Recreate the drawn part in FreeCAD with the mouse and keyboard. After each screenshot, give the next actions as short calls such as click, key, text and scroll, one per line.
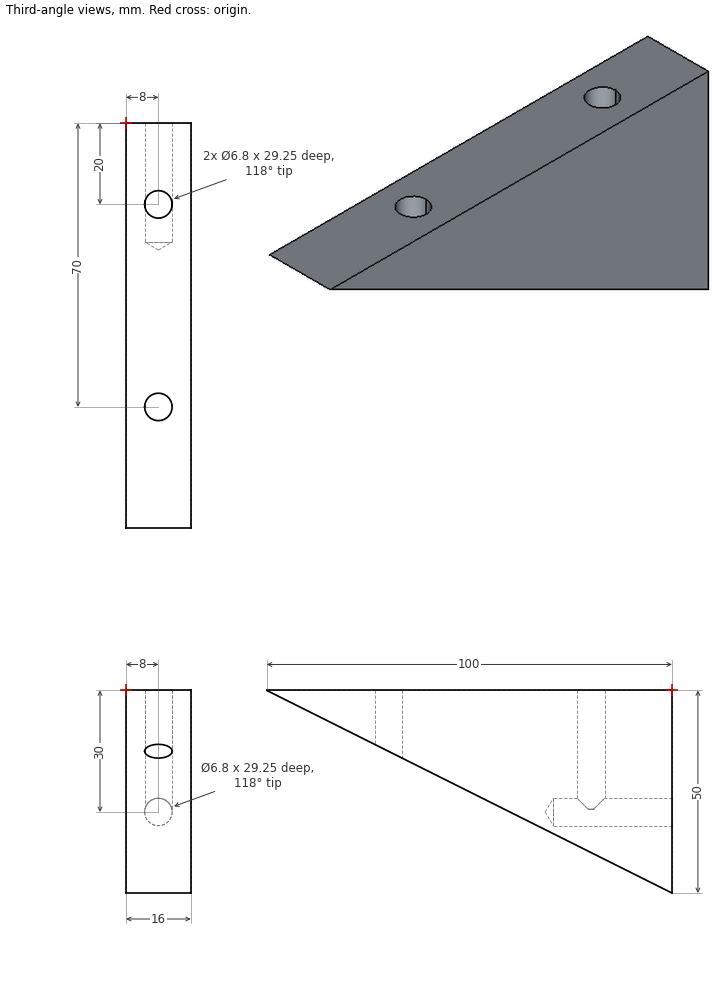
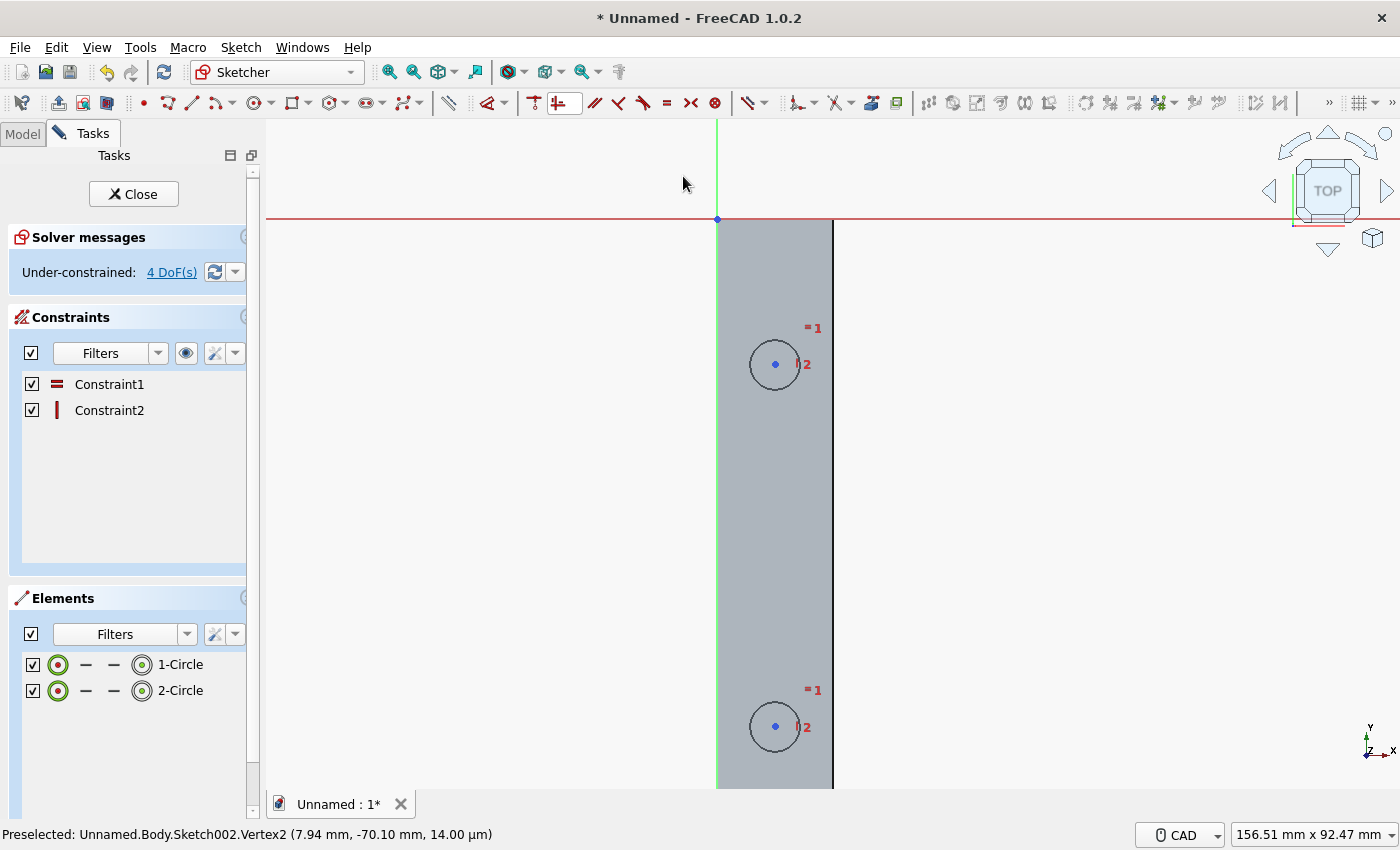
click(488, 104)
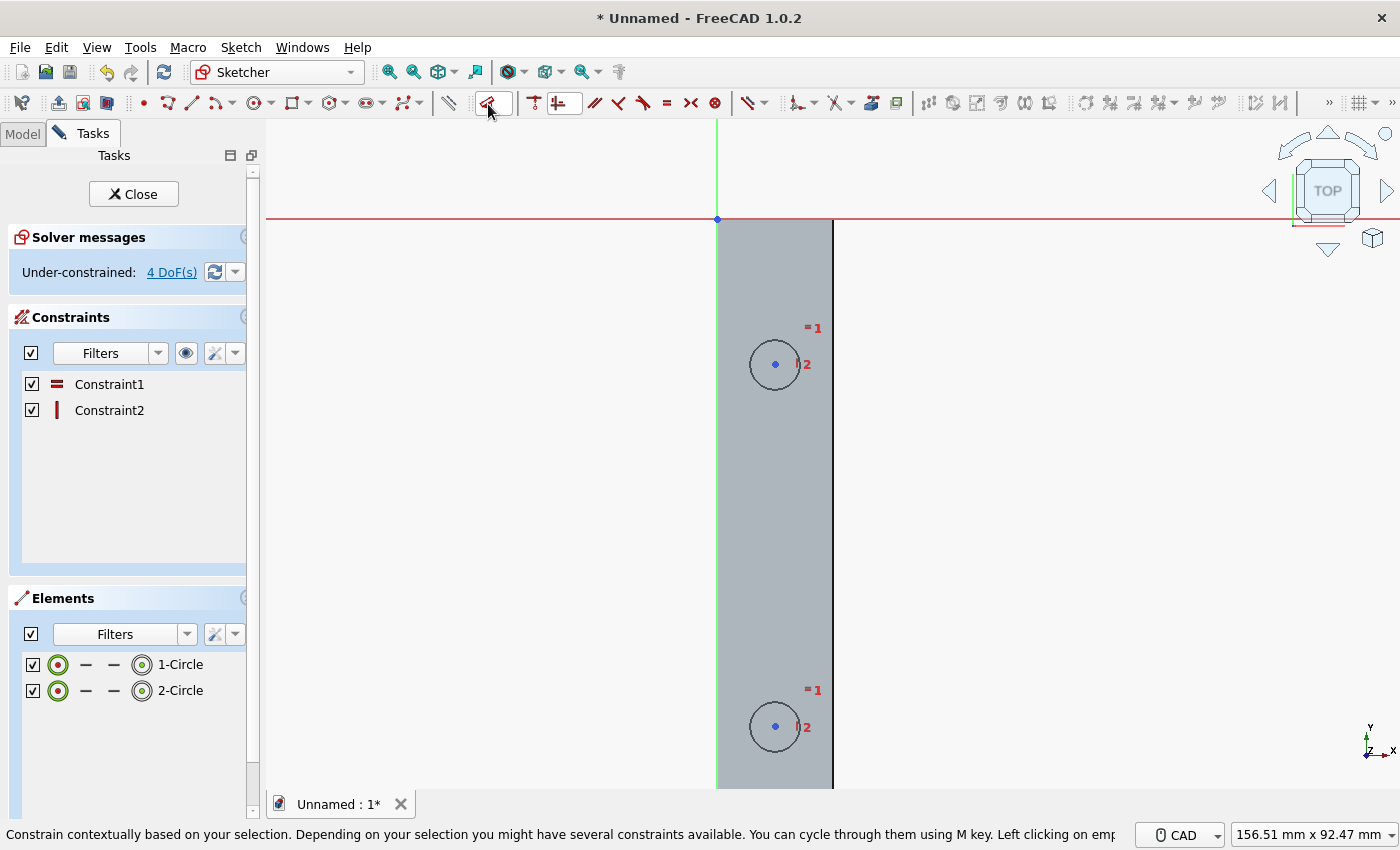
click(792, 347)
click(814, 324)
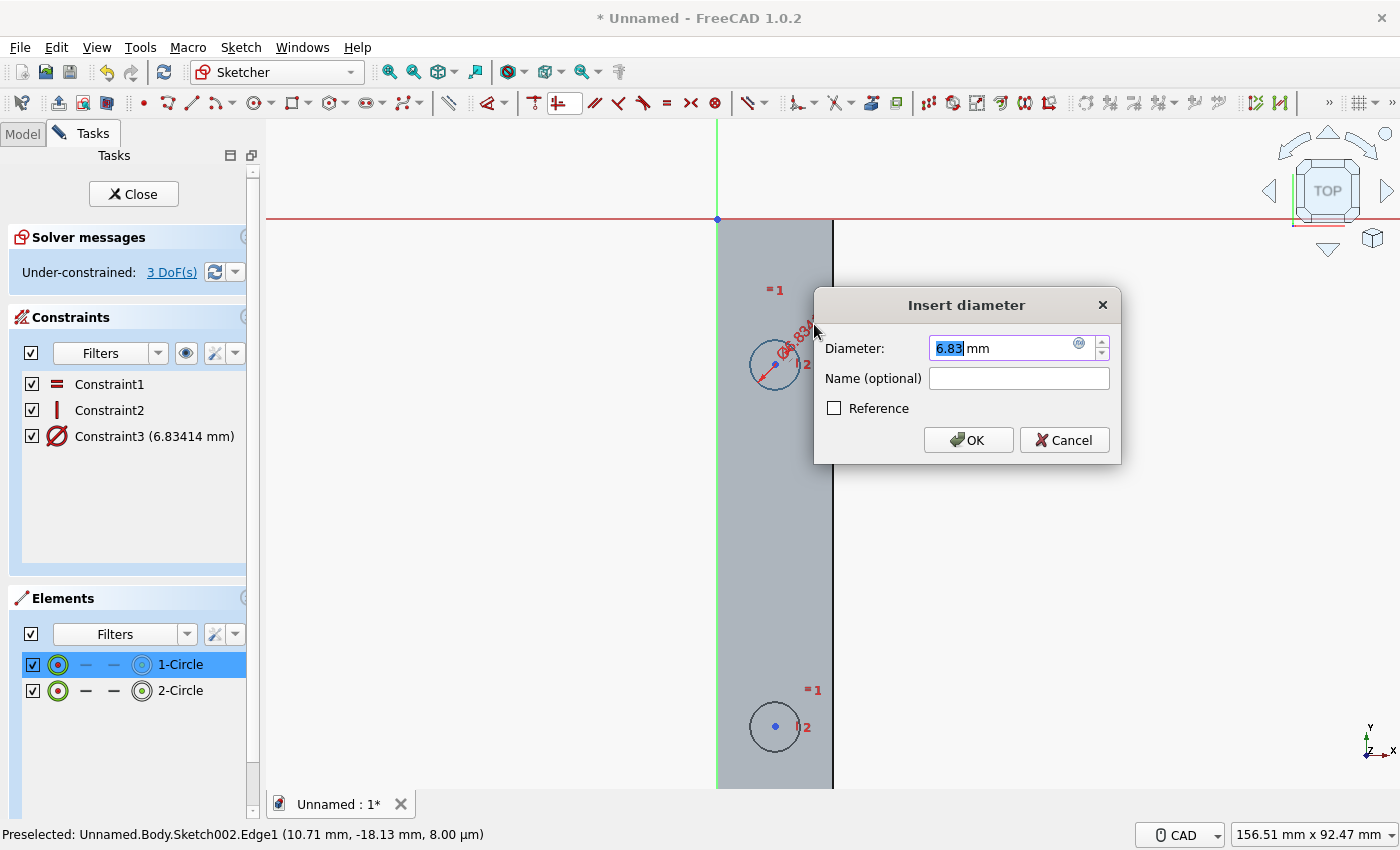
text(6.8)
key(Return)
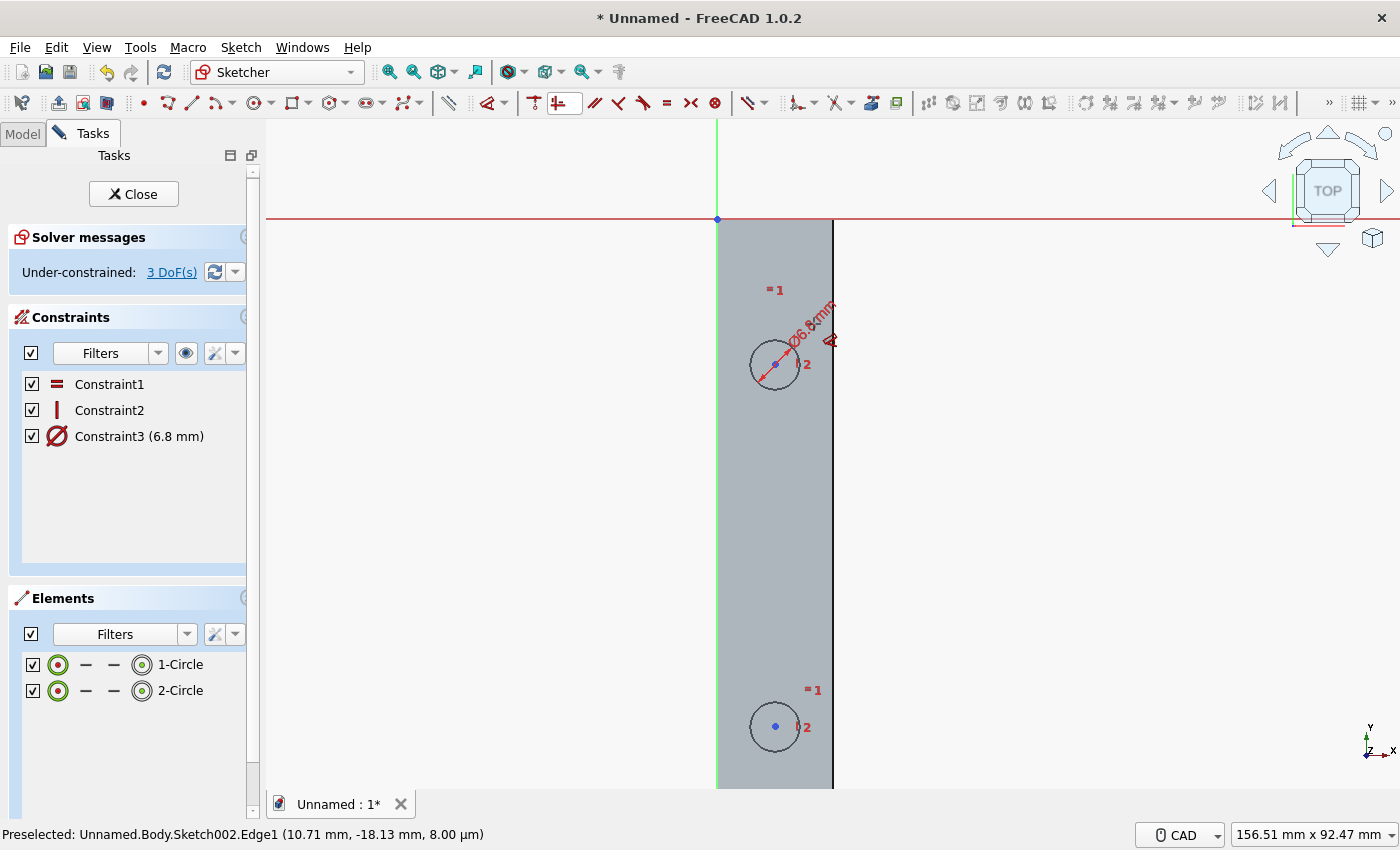
click(775, 365)
click(746, 185)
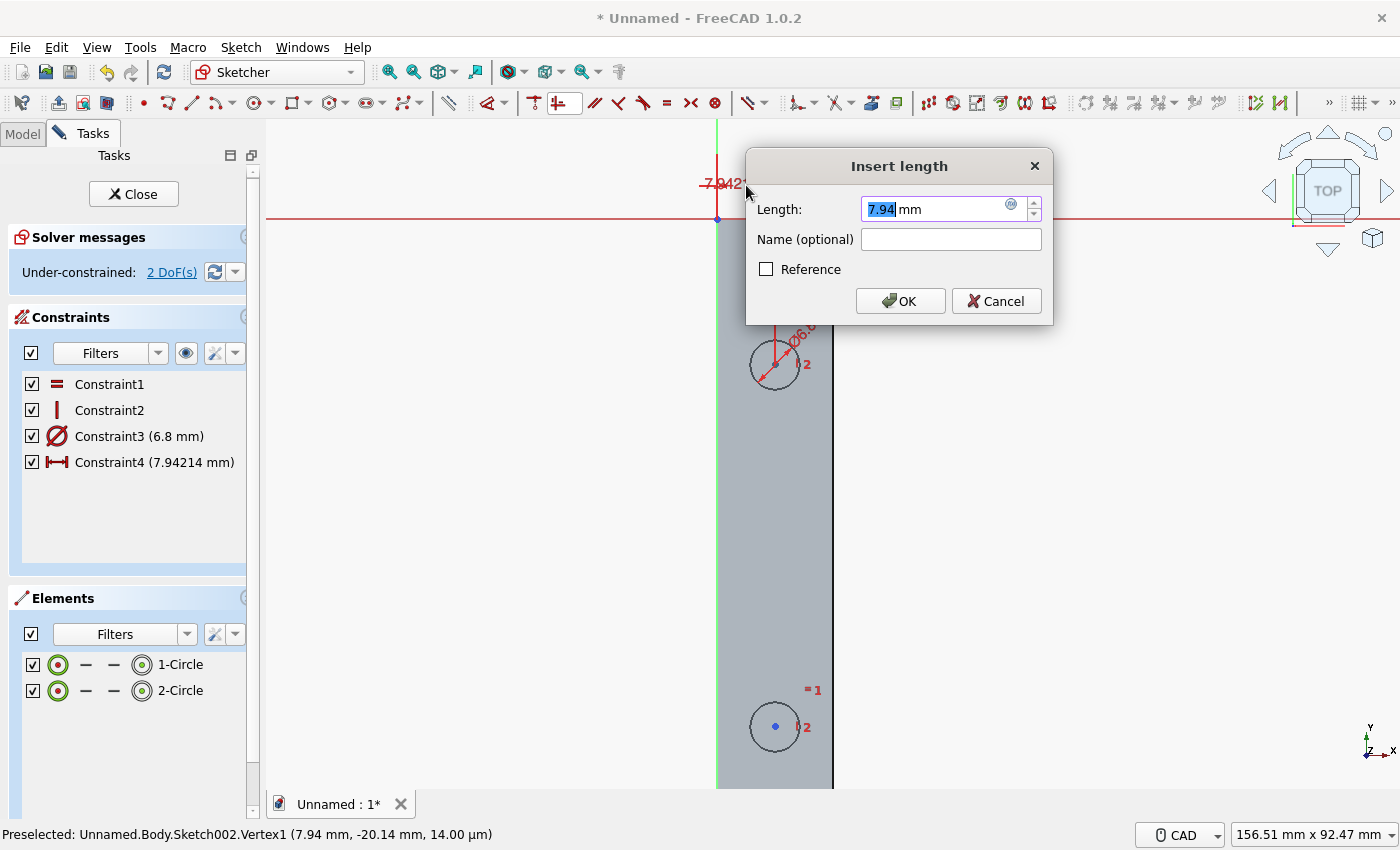
text(8)
key(Return)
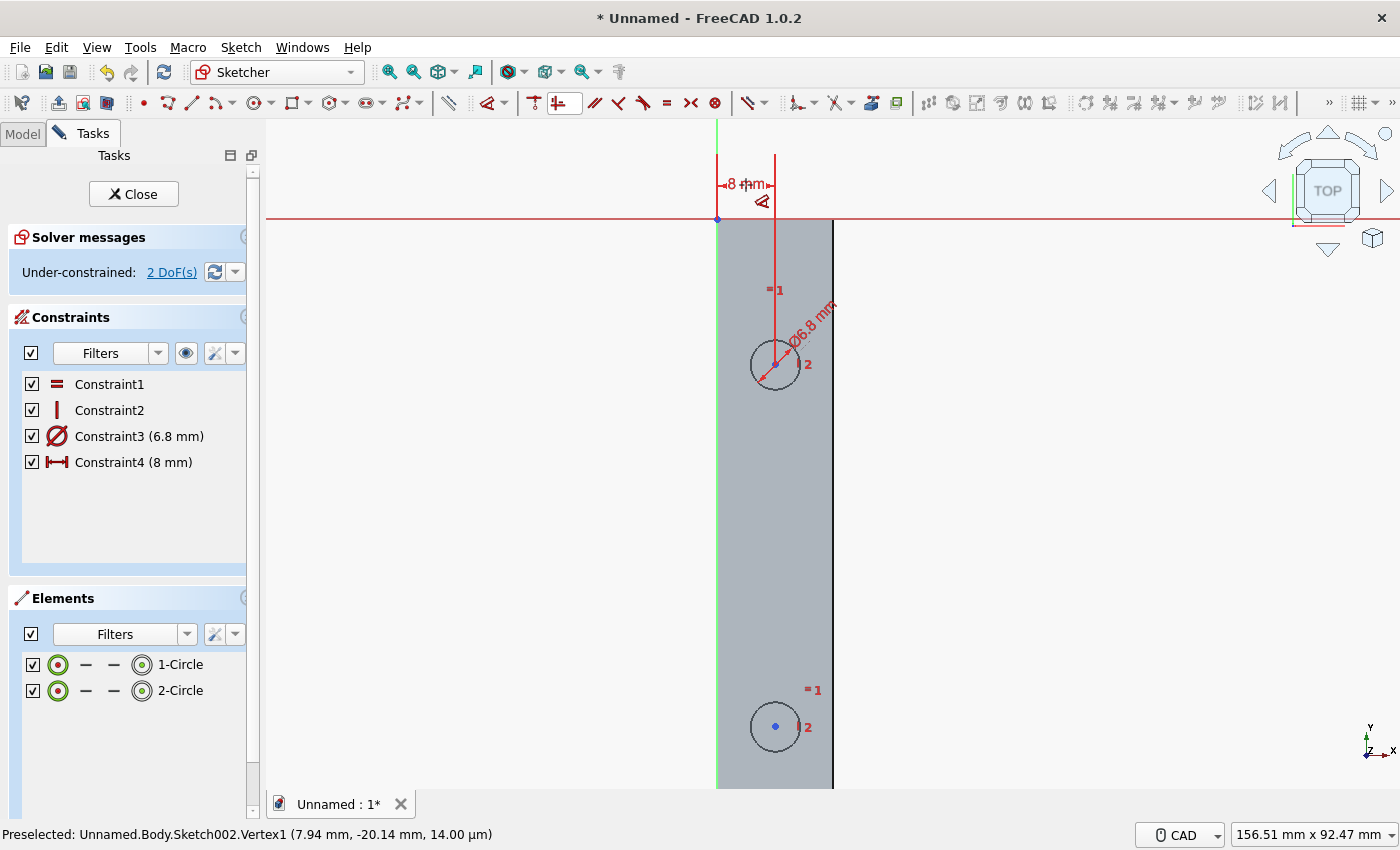
click(775, 365)
click(683, 292)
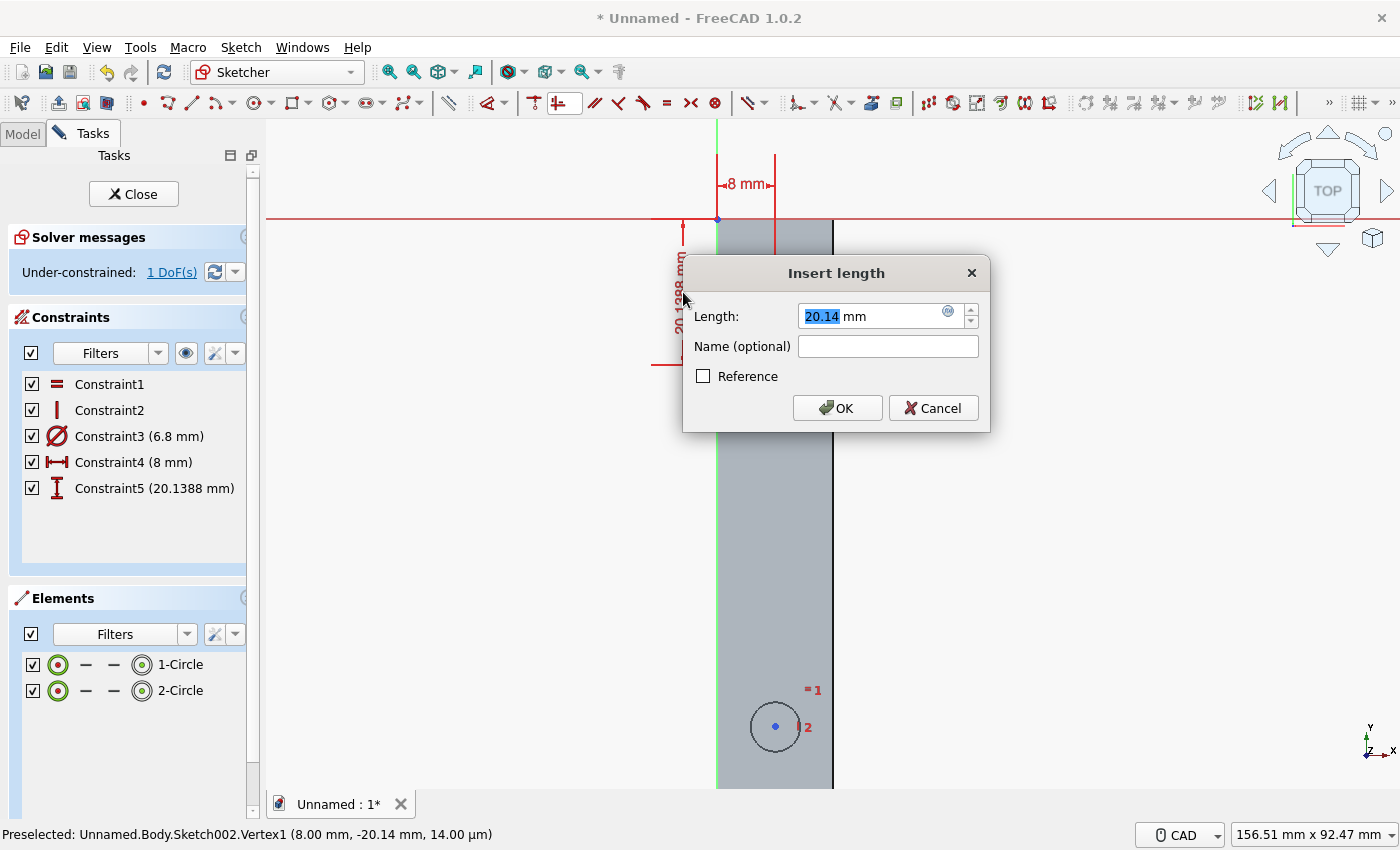
text(20)
key(Return)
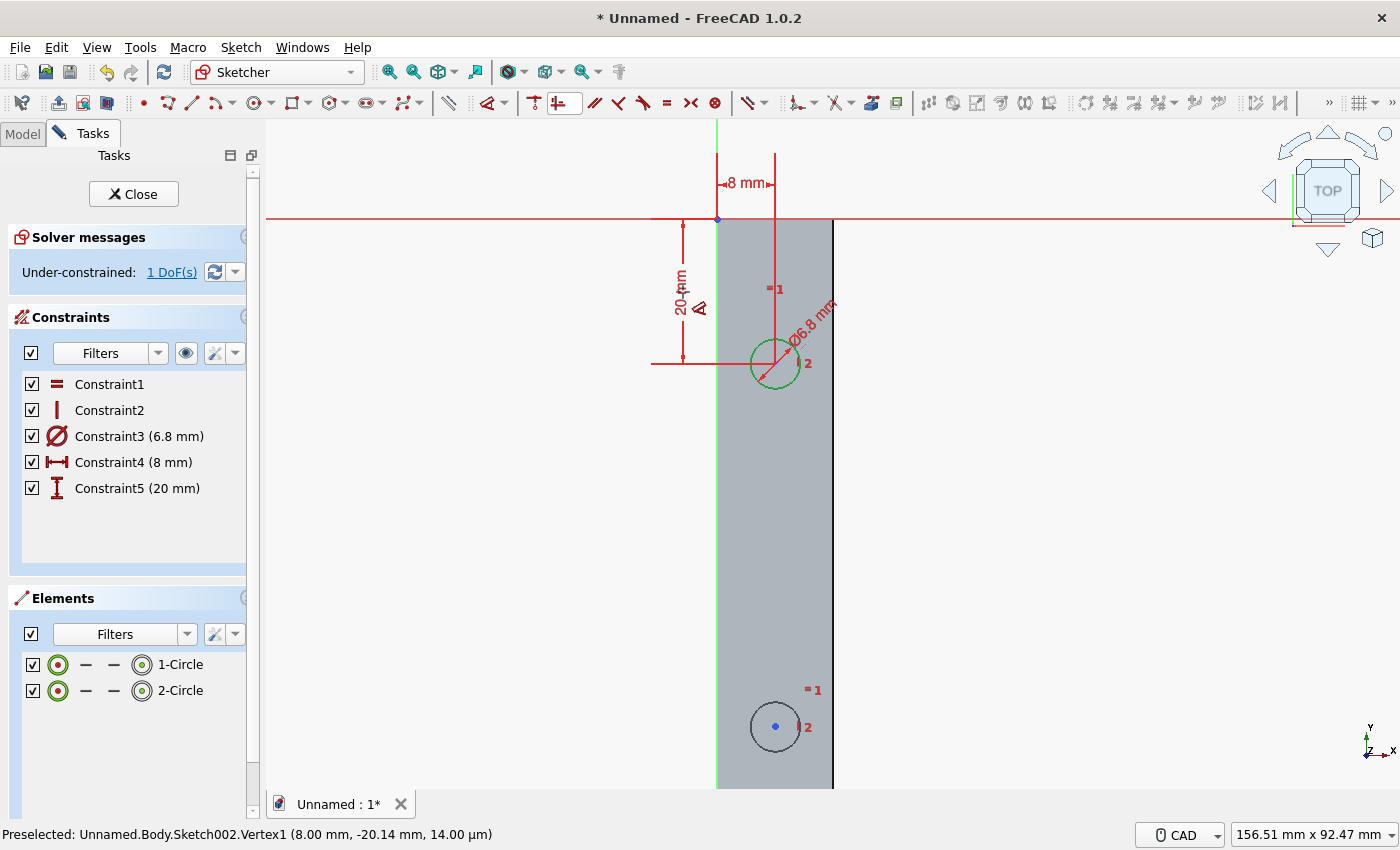
click(775, 727)
click(683, 473)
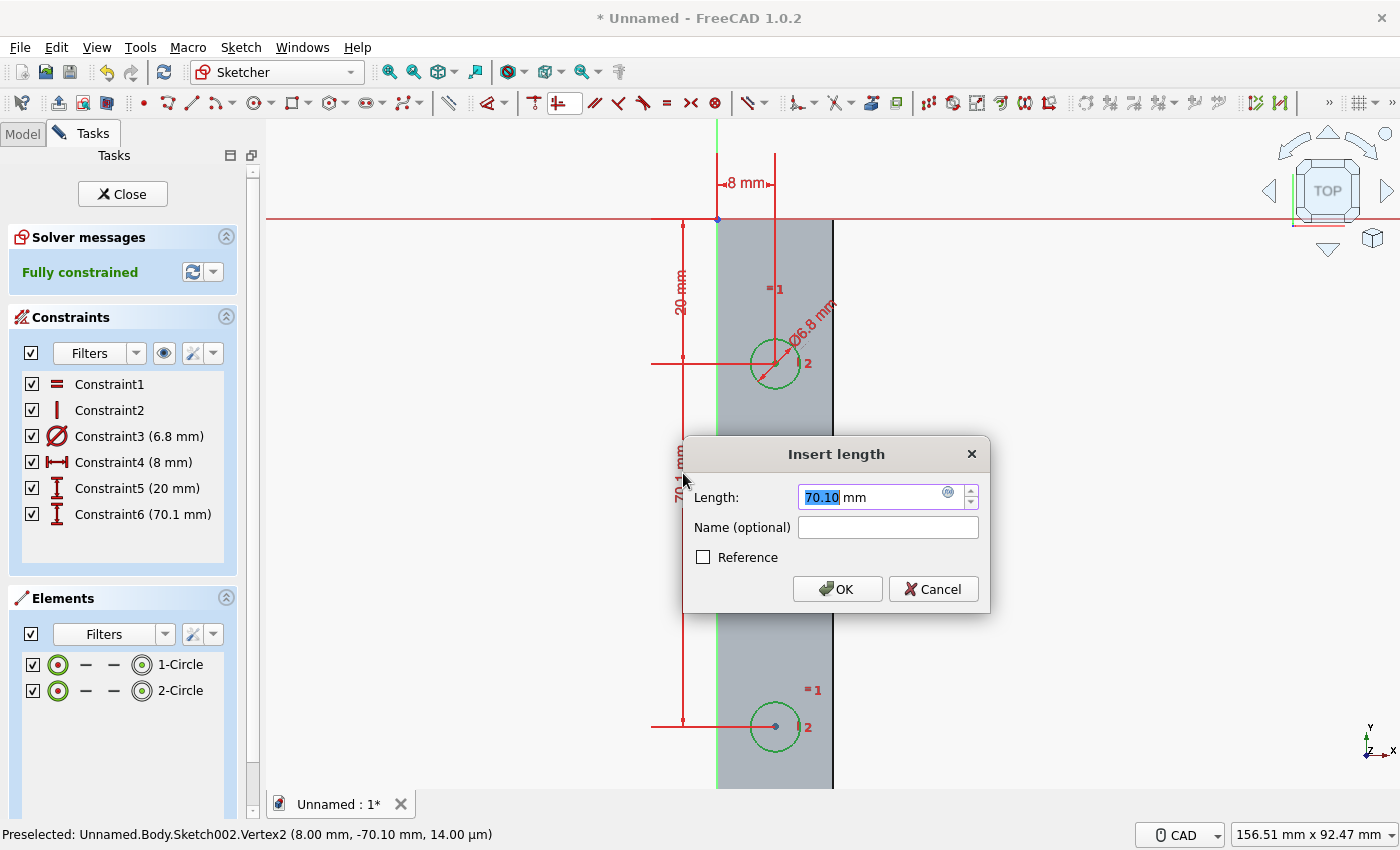
text(70)
key(Return)
key(Escape)